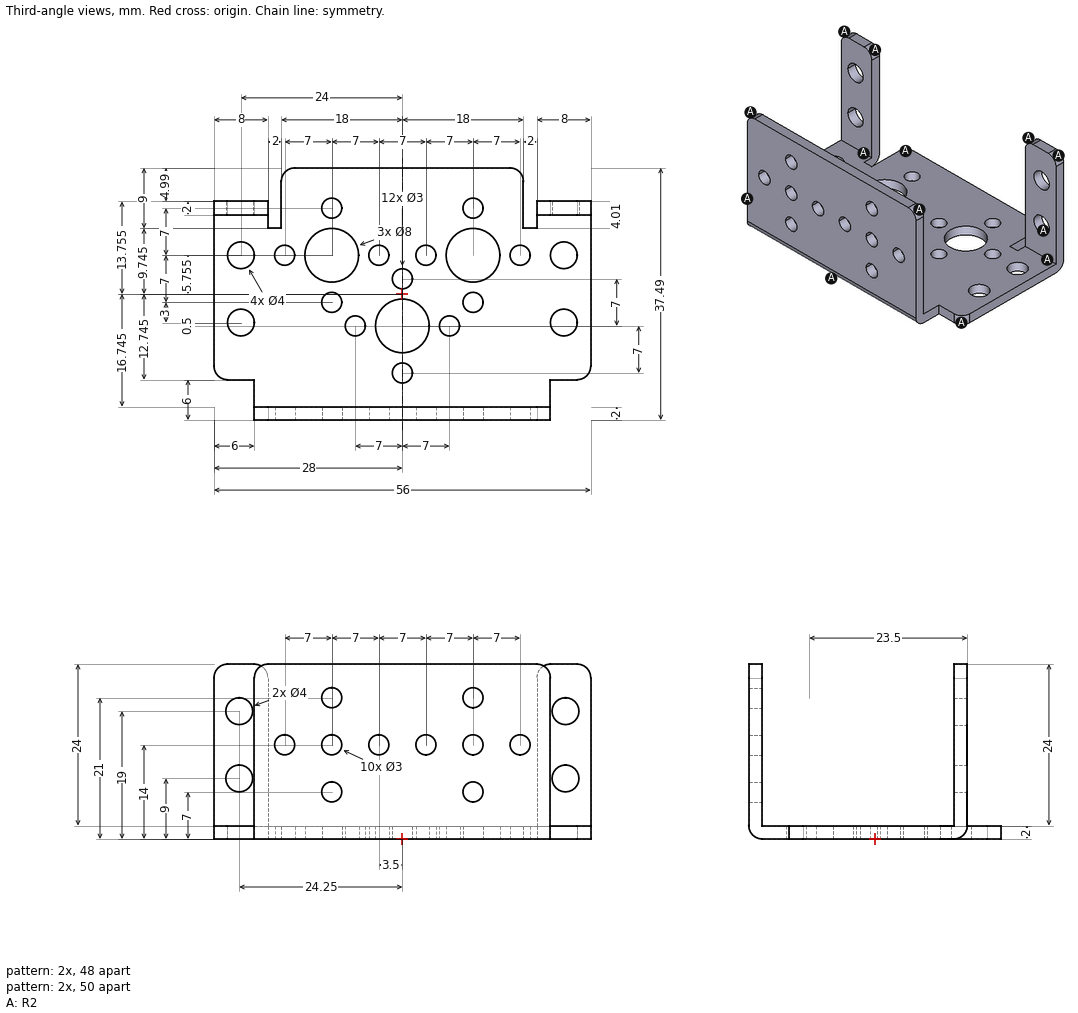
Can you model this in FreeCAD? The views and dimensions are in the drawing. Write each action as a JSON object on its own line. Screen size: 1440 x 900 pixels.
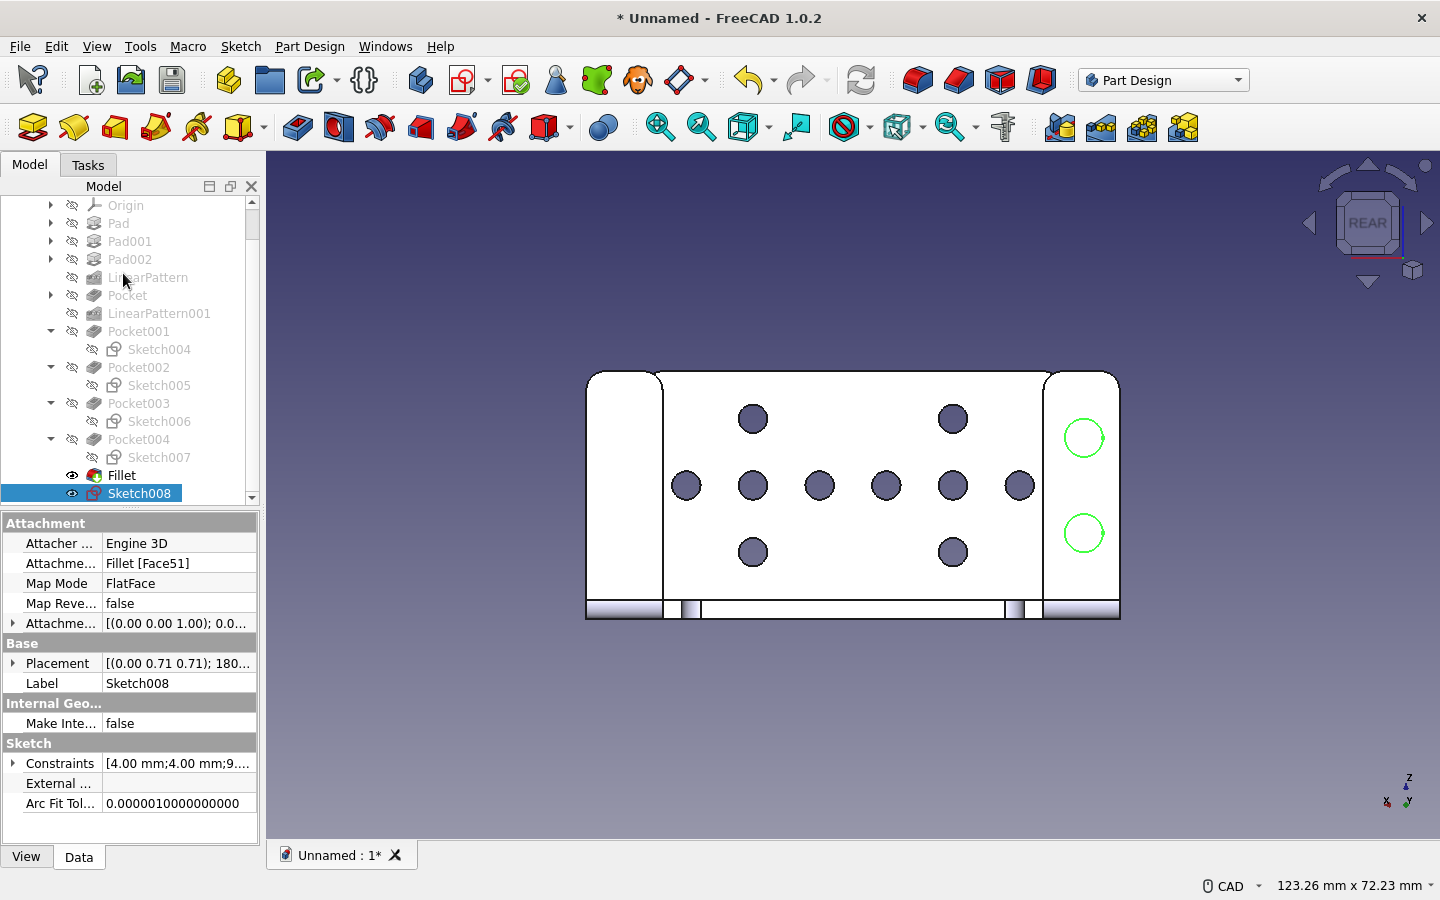
{"action": "left_click", "coordinate": [298, 128]}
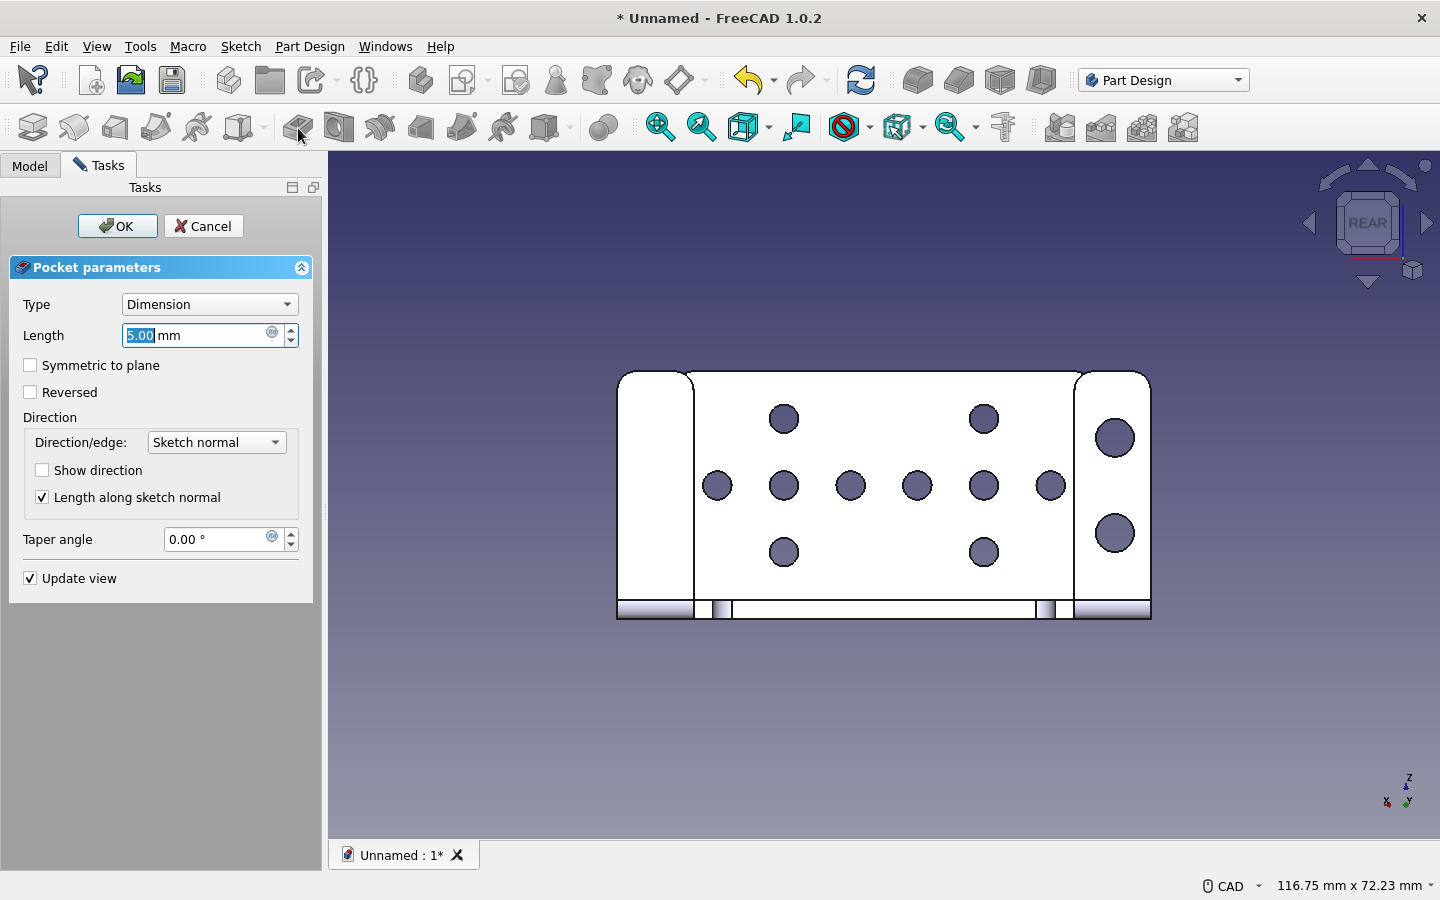
{"action": "type", "text": "23.5"}
{"action": "key", "text": "Tab"}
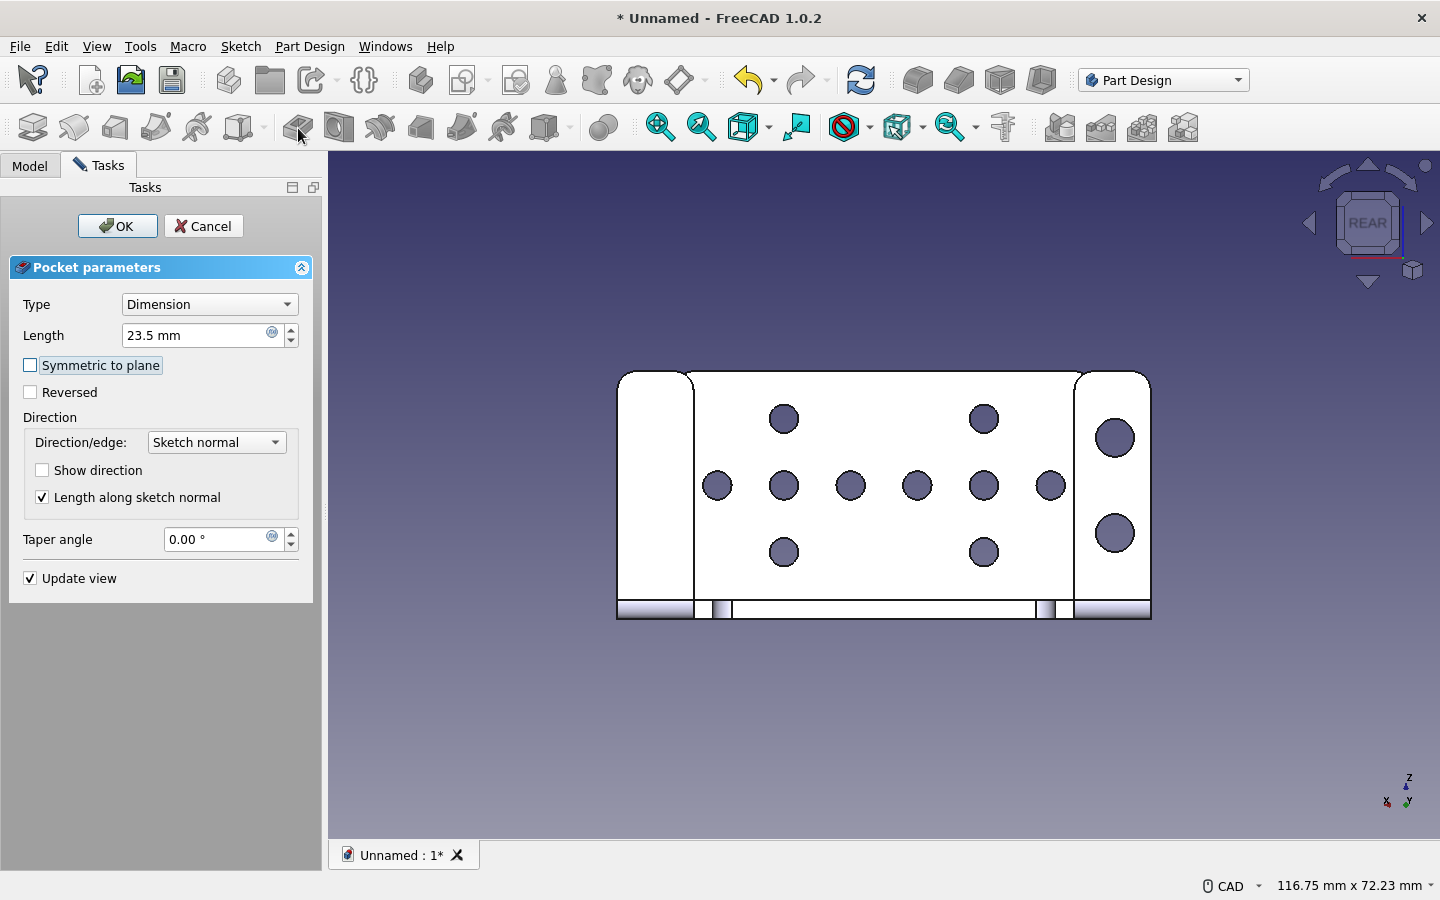
{"action": "left_click", "coordinate": [118, 226]}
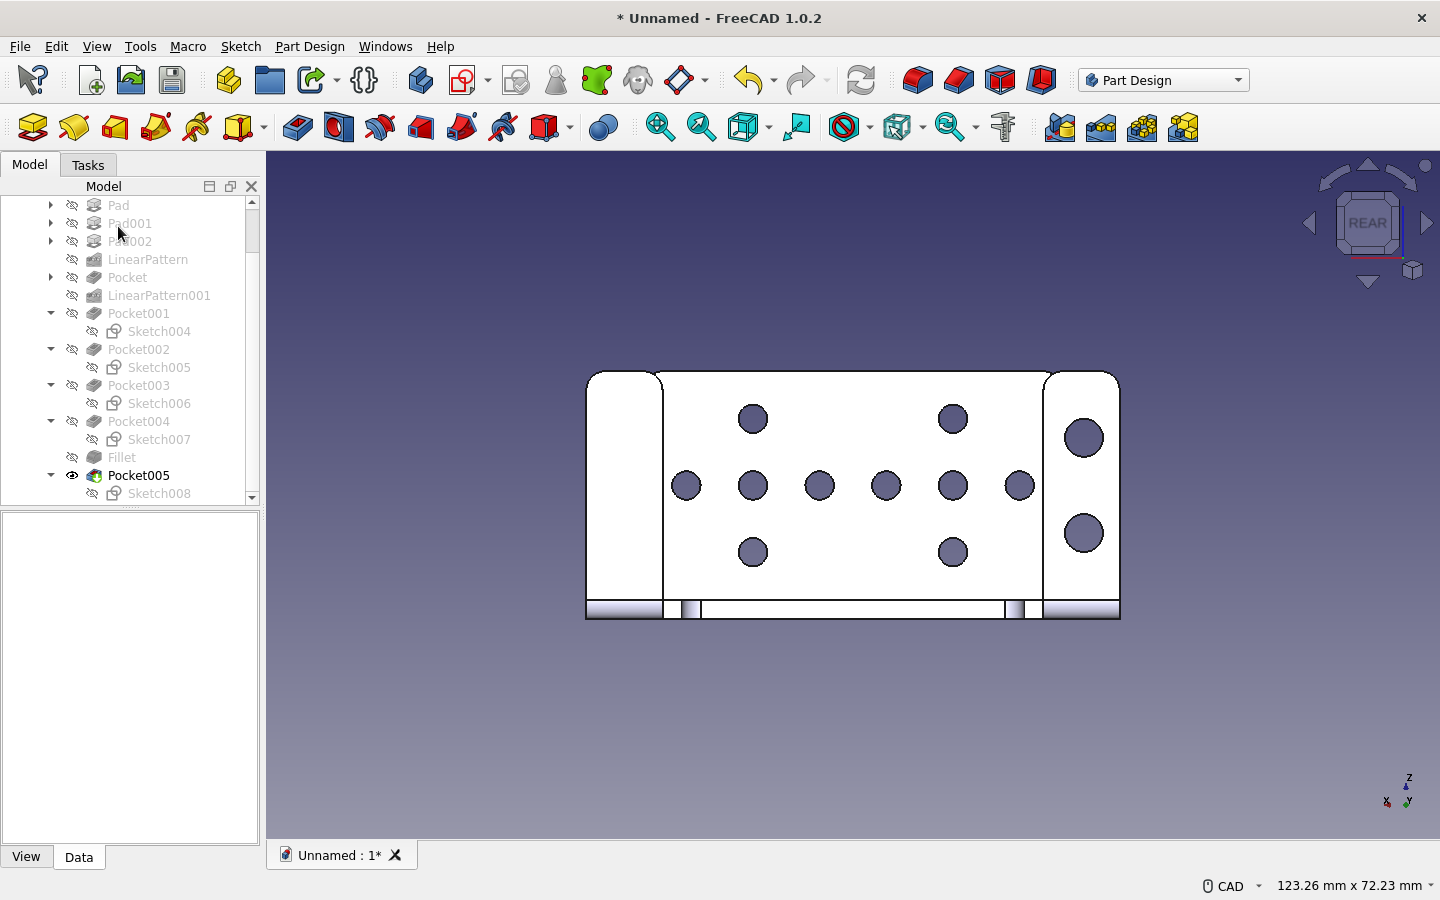
{"action": "left_click", "coordinate": [117, 475]}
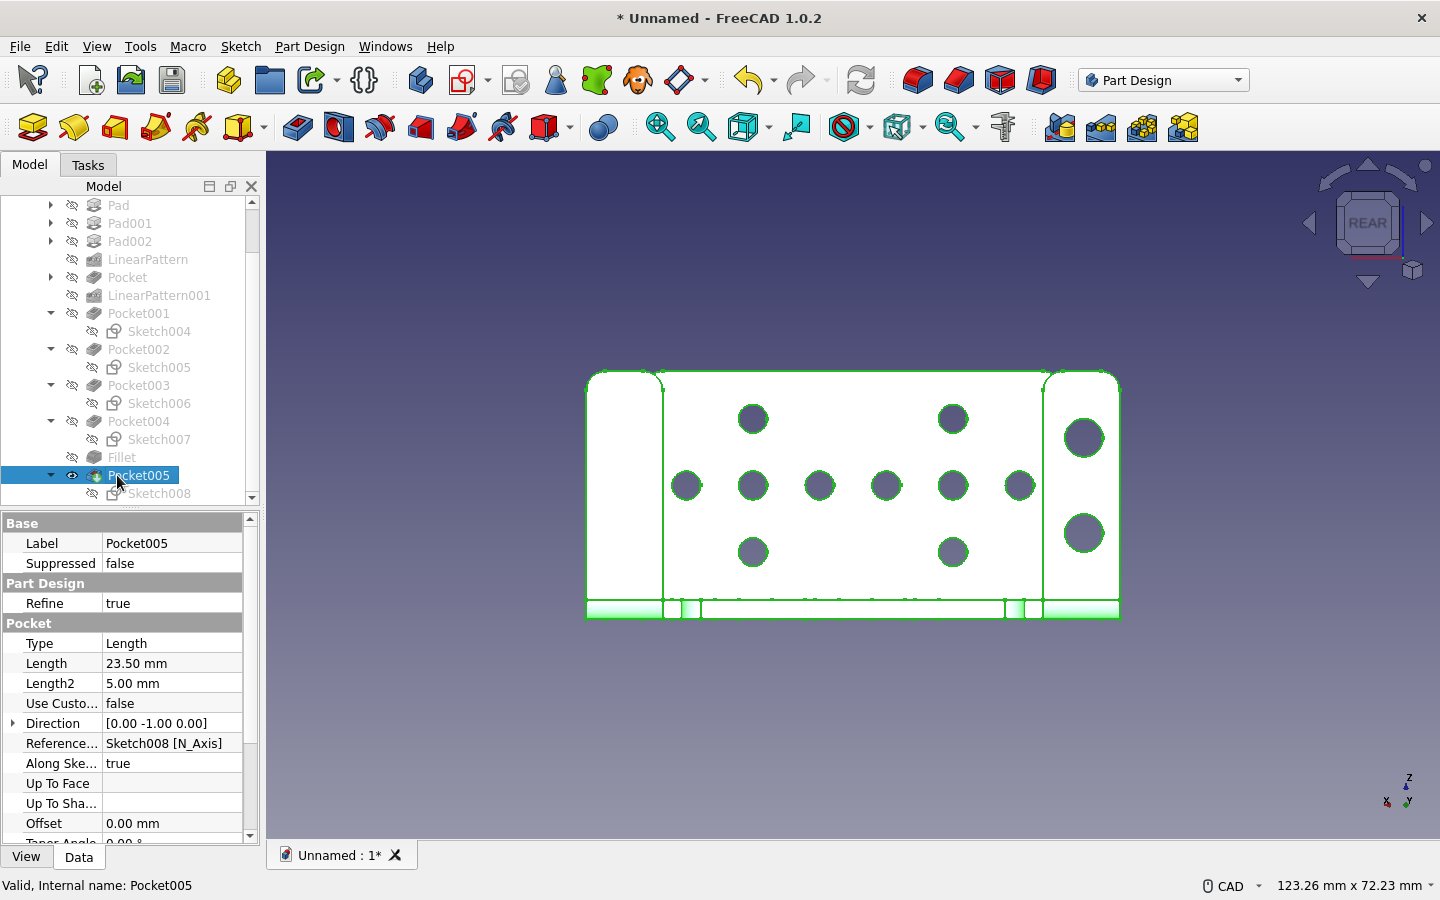
{"action": "left_click", "coordinate": [1060, 128]}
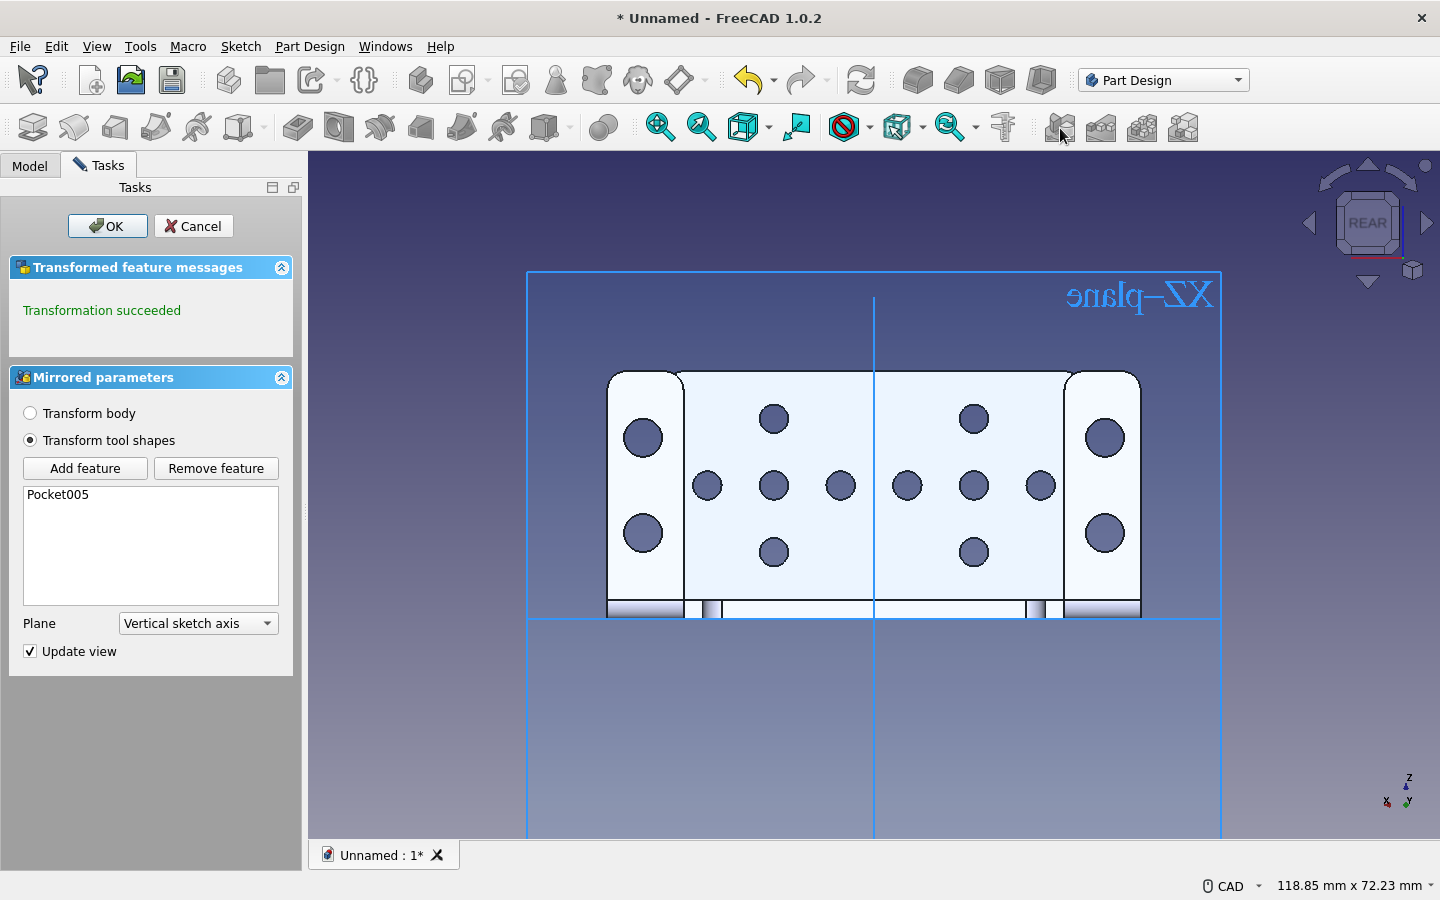
{"action": "left_click", "coordinate": [199, 624]}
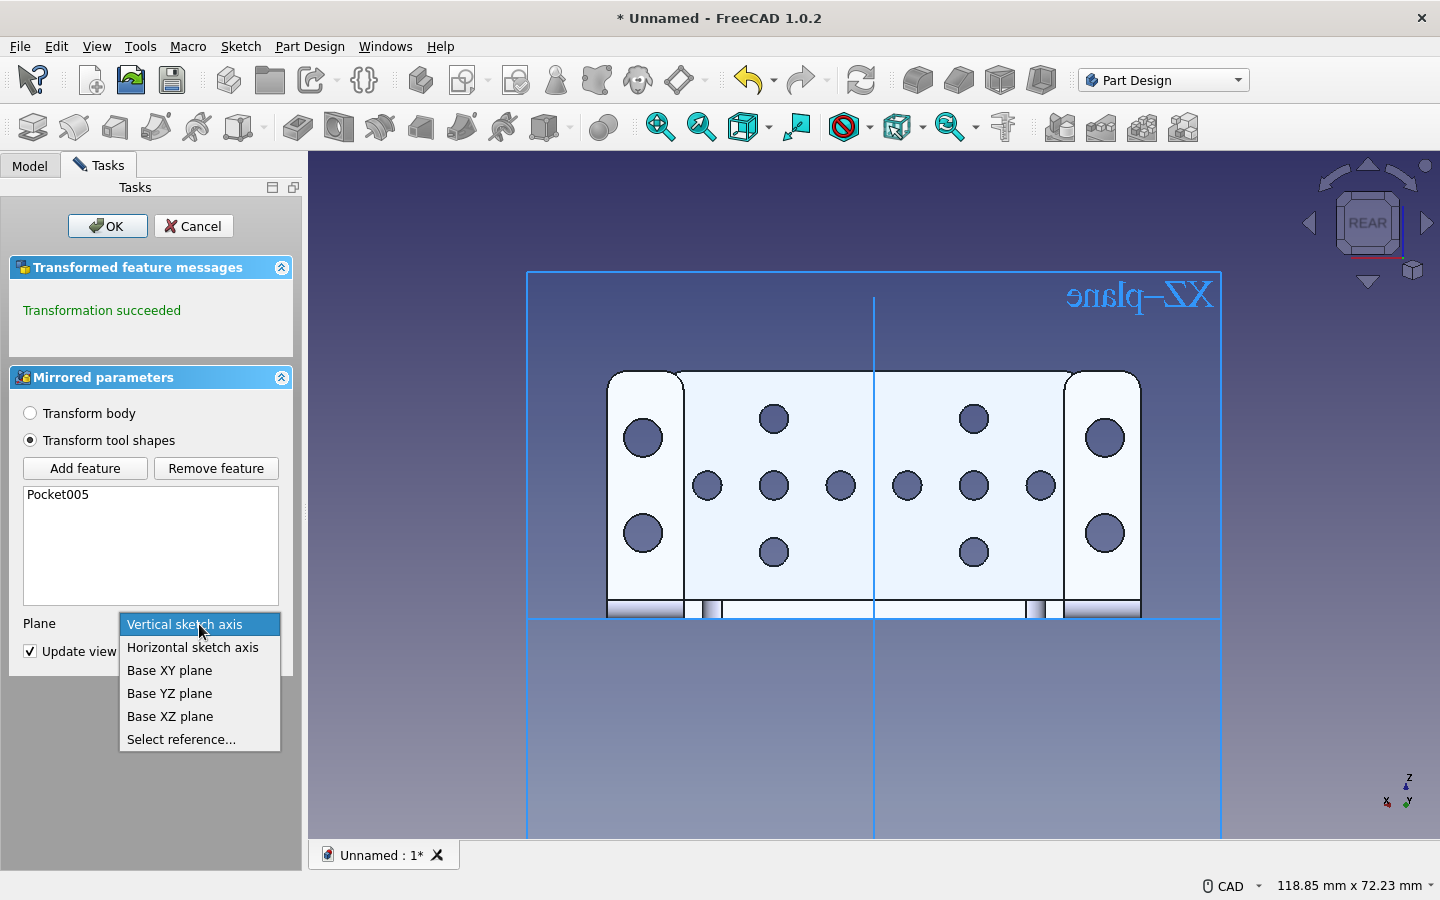
{"action": "left_click", "coordinate": [198, 694]}